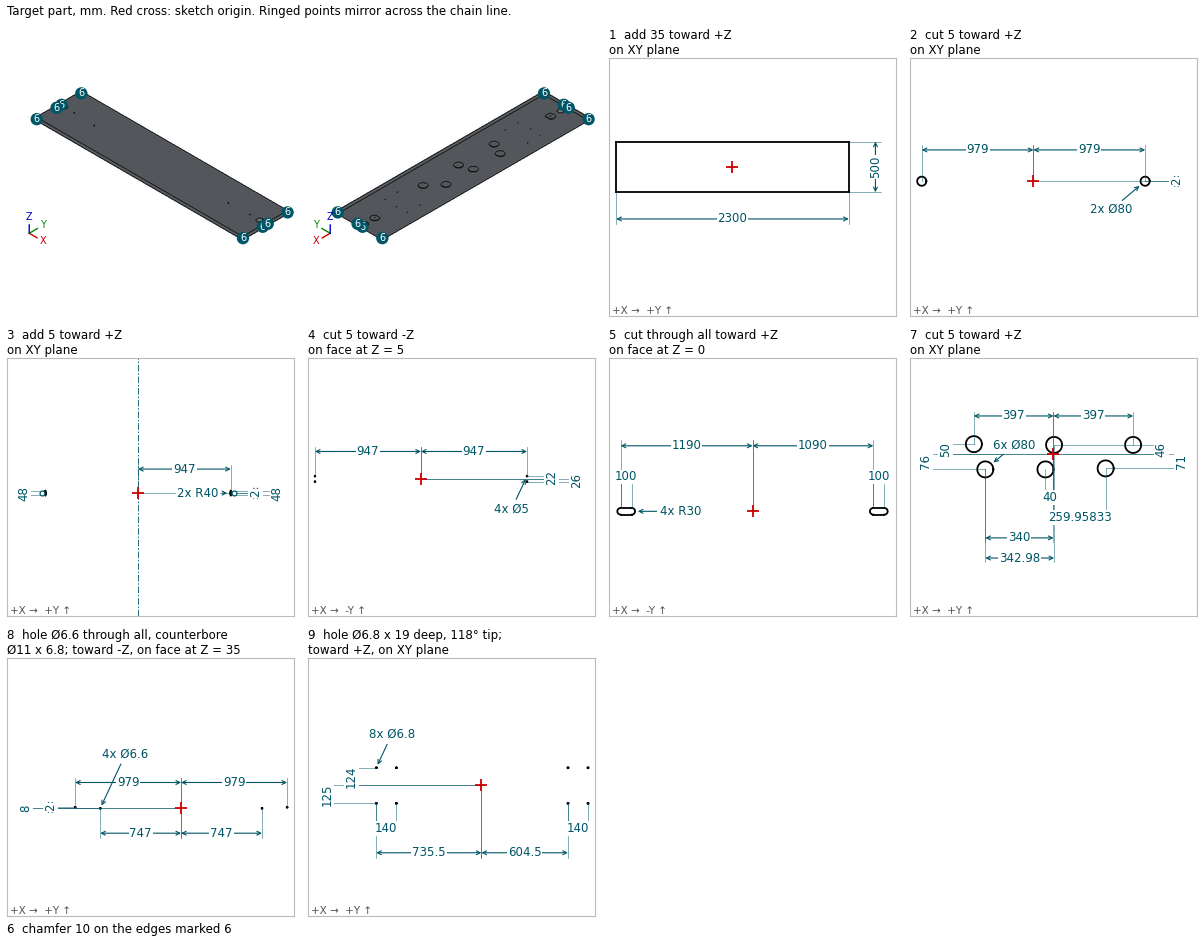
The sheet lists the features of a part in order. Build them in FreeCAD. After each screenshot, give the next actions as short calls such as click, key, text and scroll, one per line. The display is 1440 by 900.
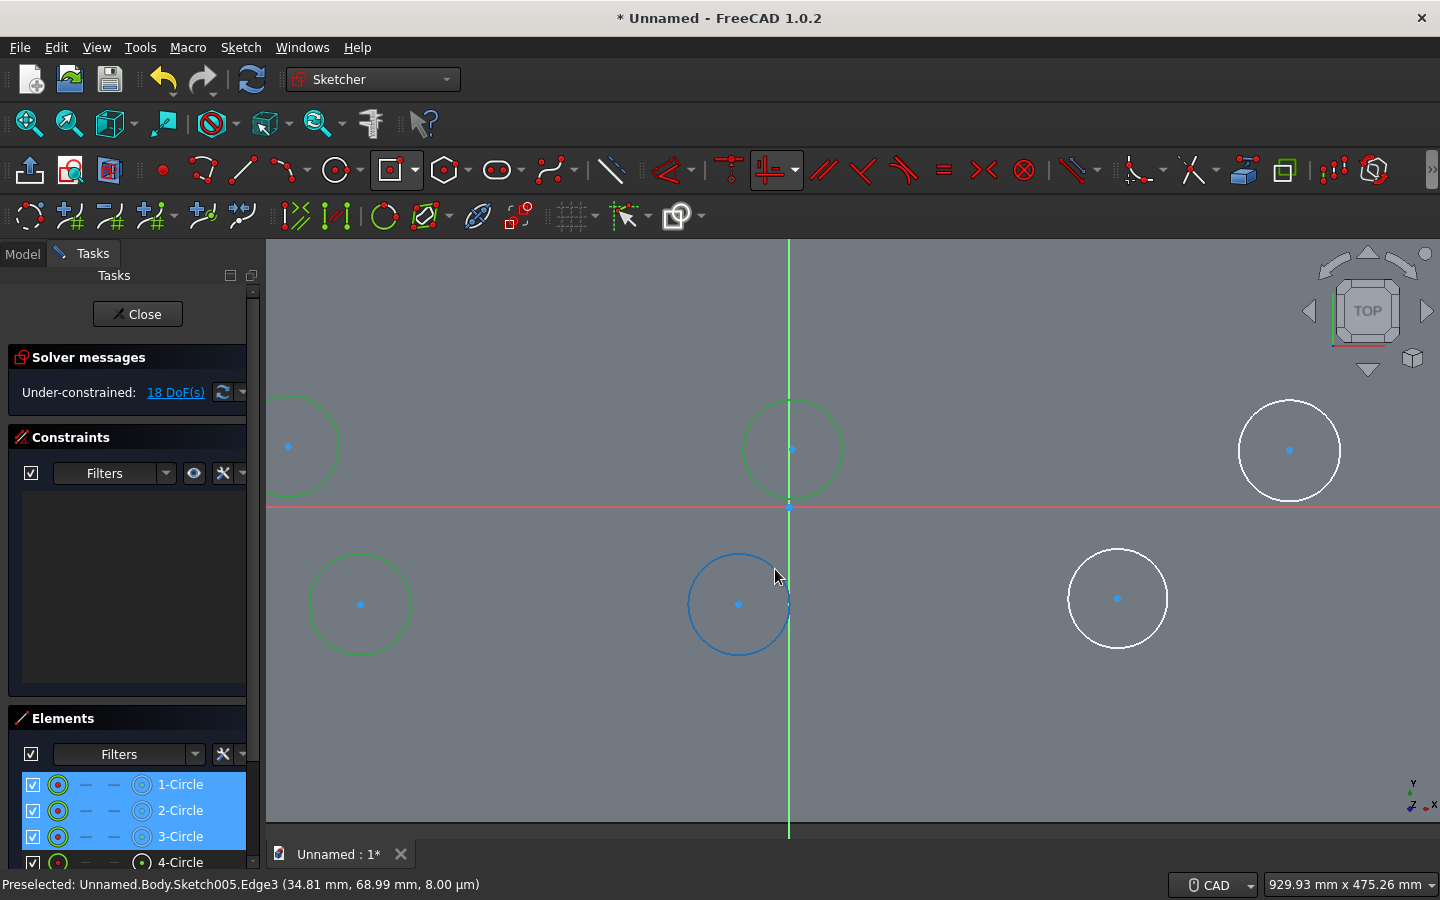
click(775, 569)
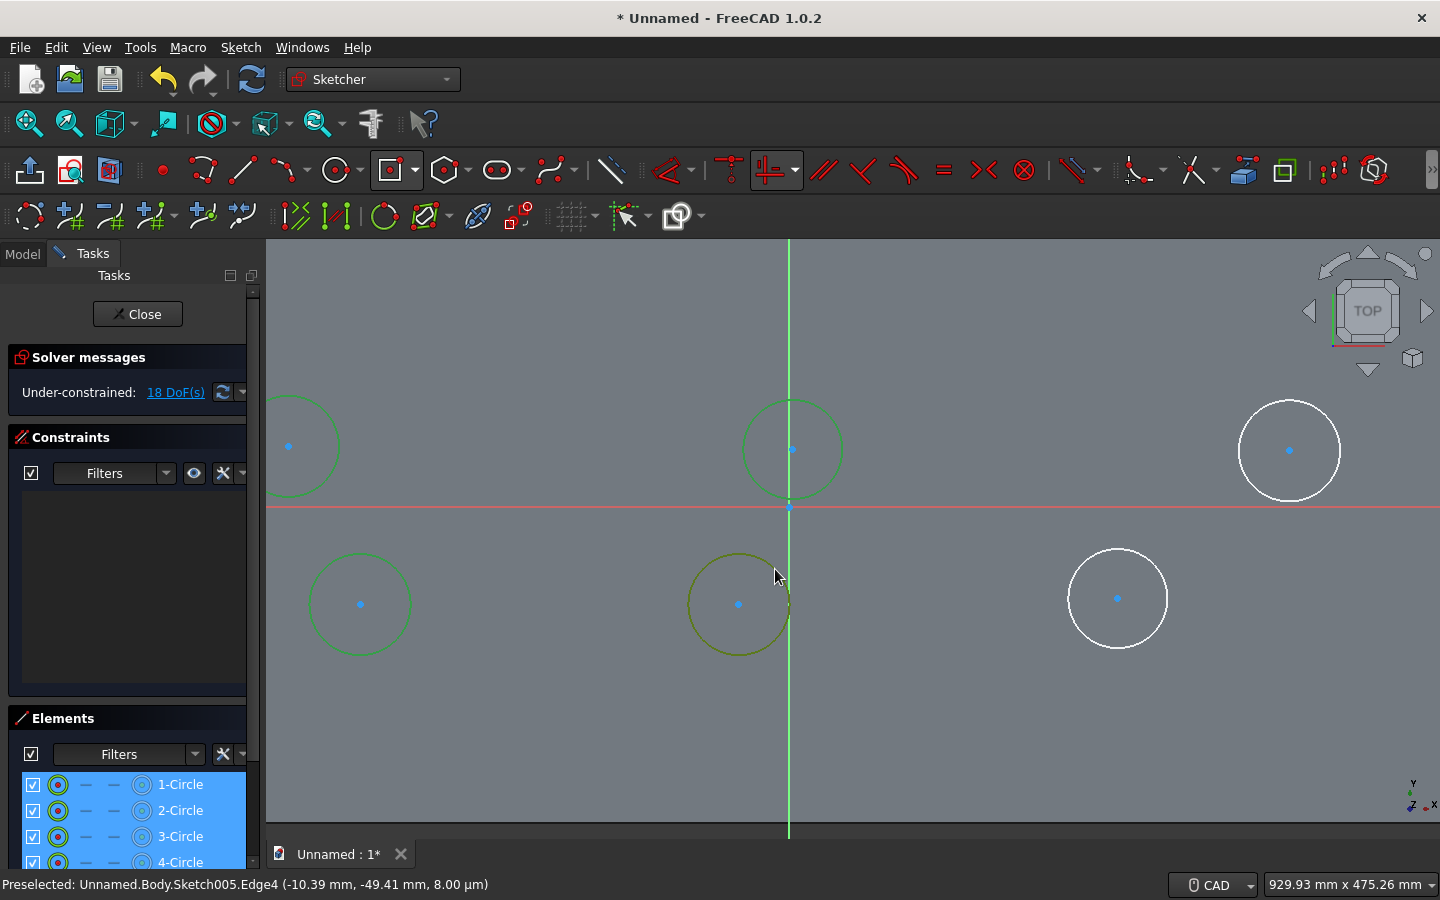
click(1153, 563)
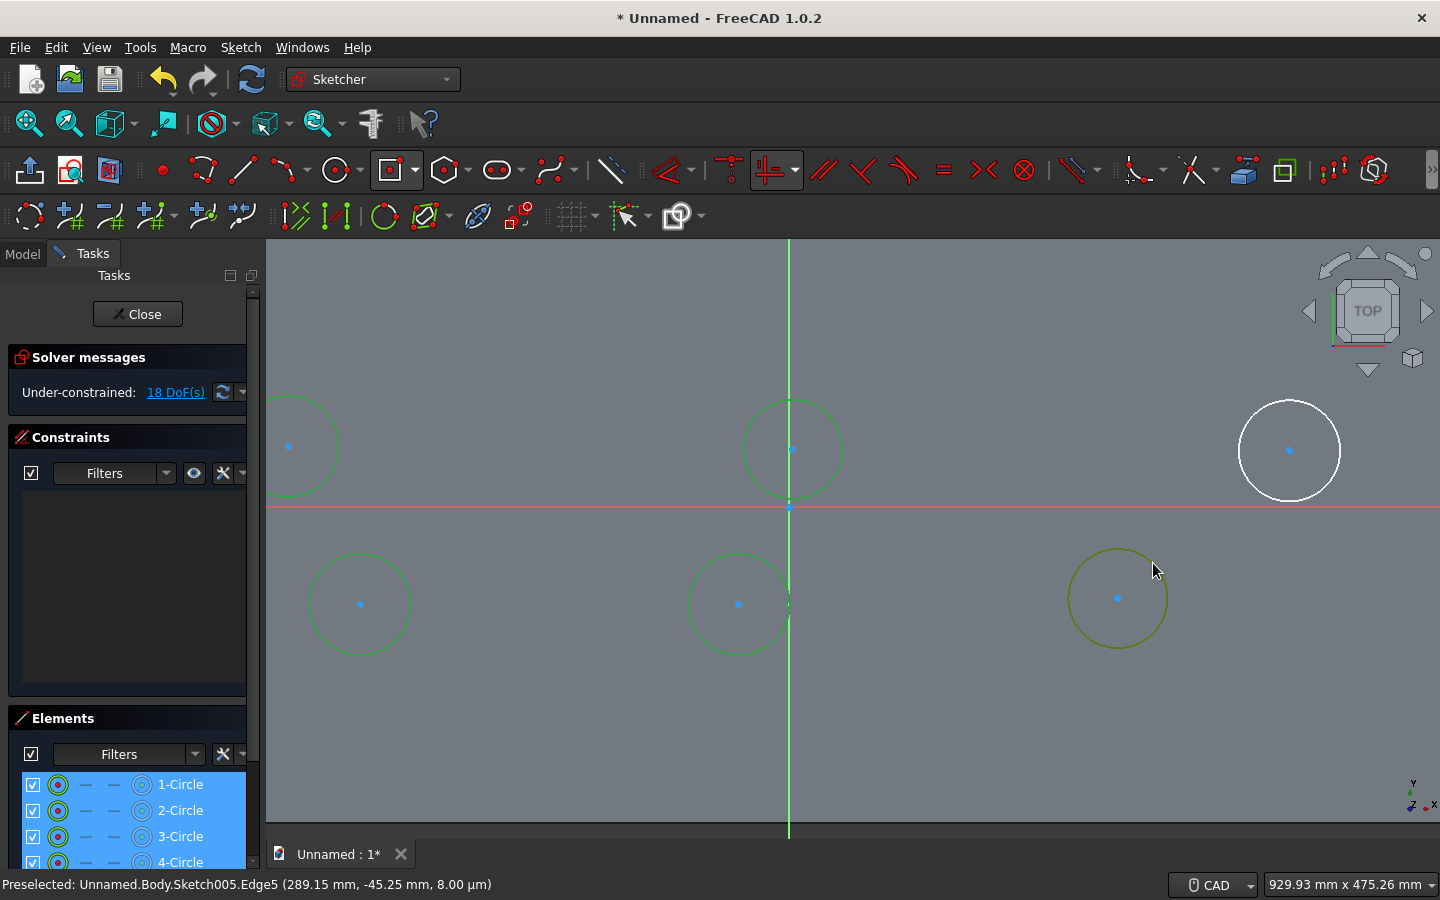
click(1254, 415)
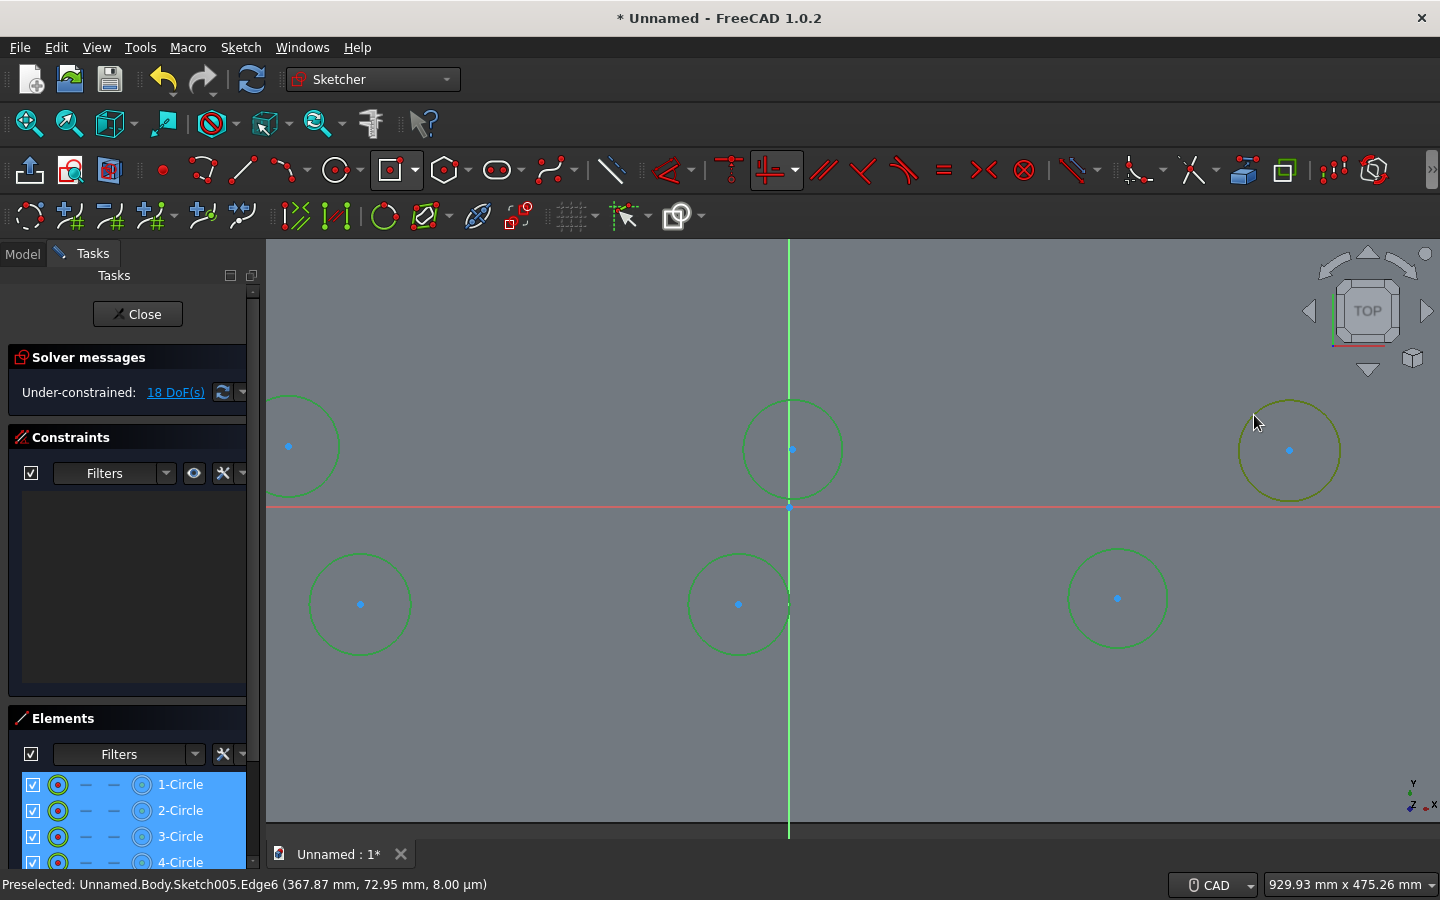
key(e)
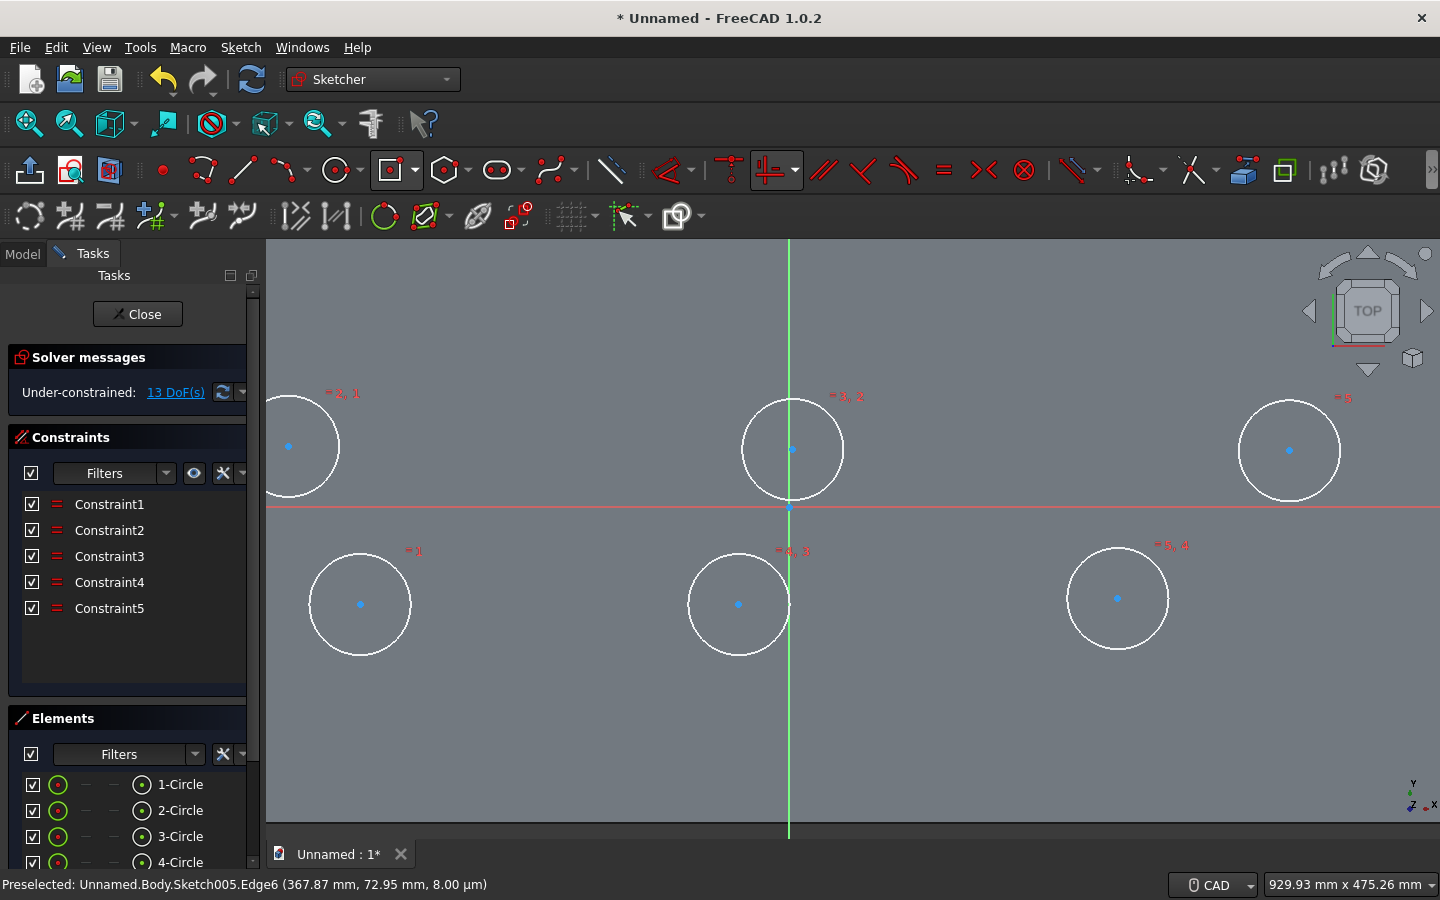
click(360, 605)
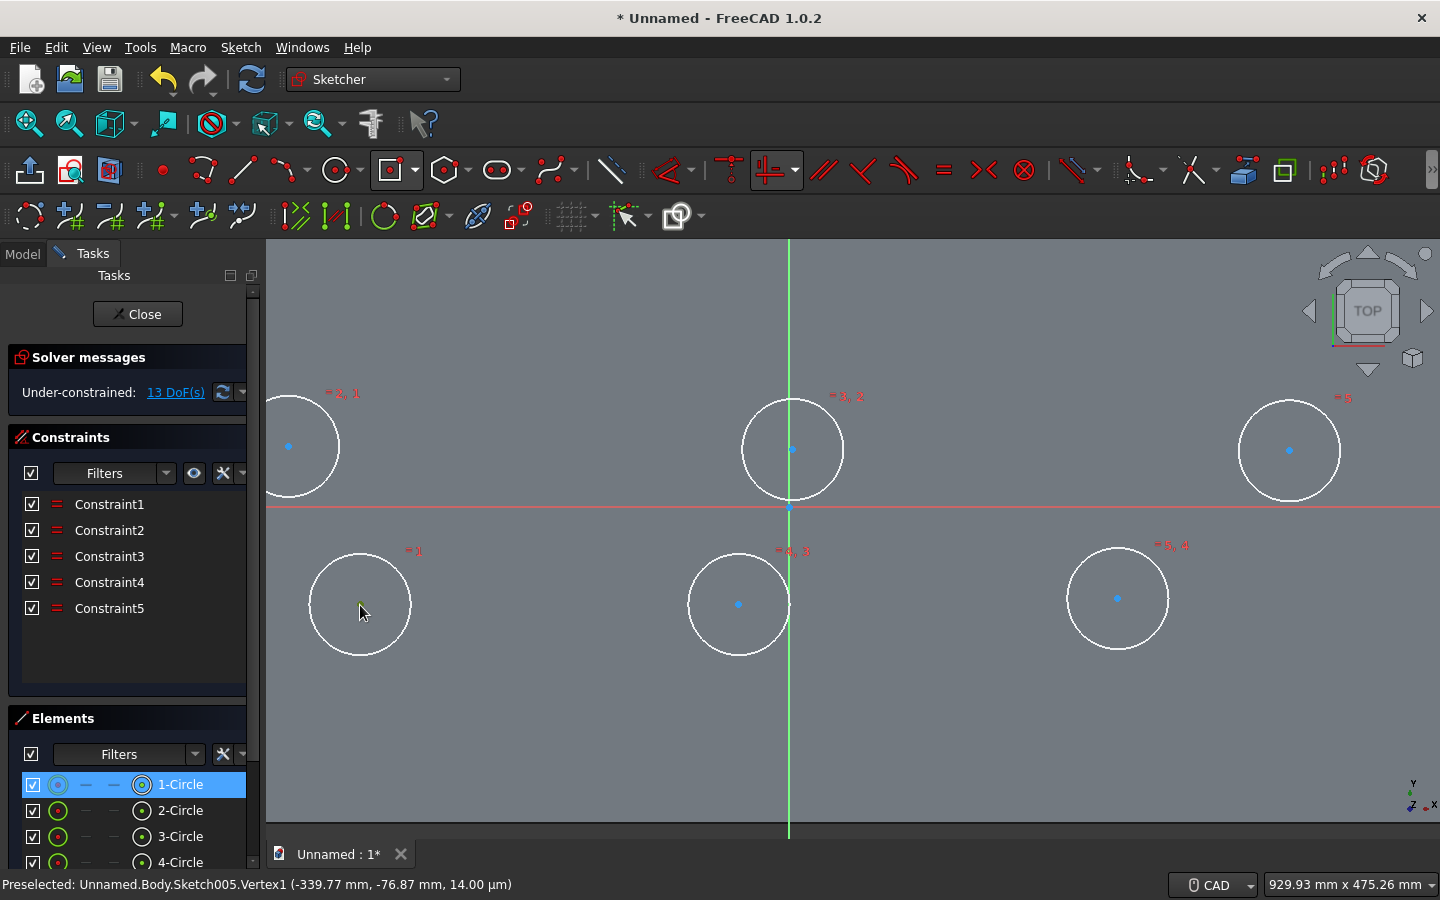
click(739, 605)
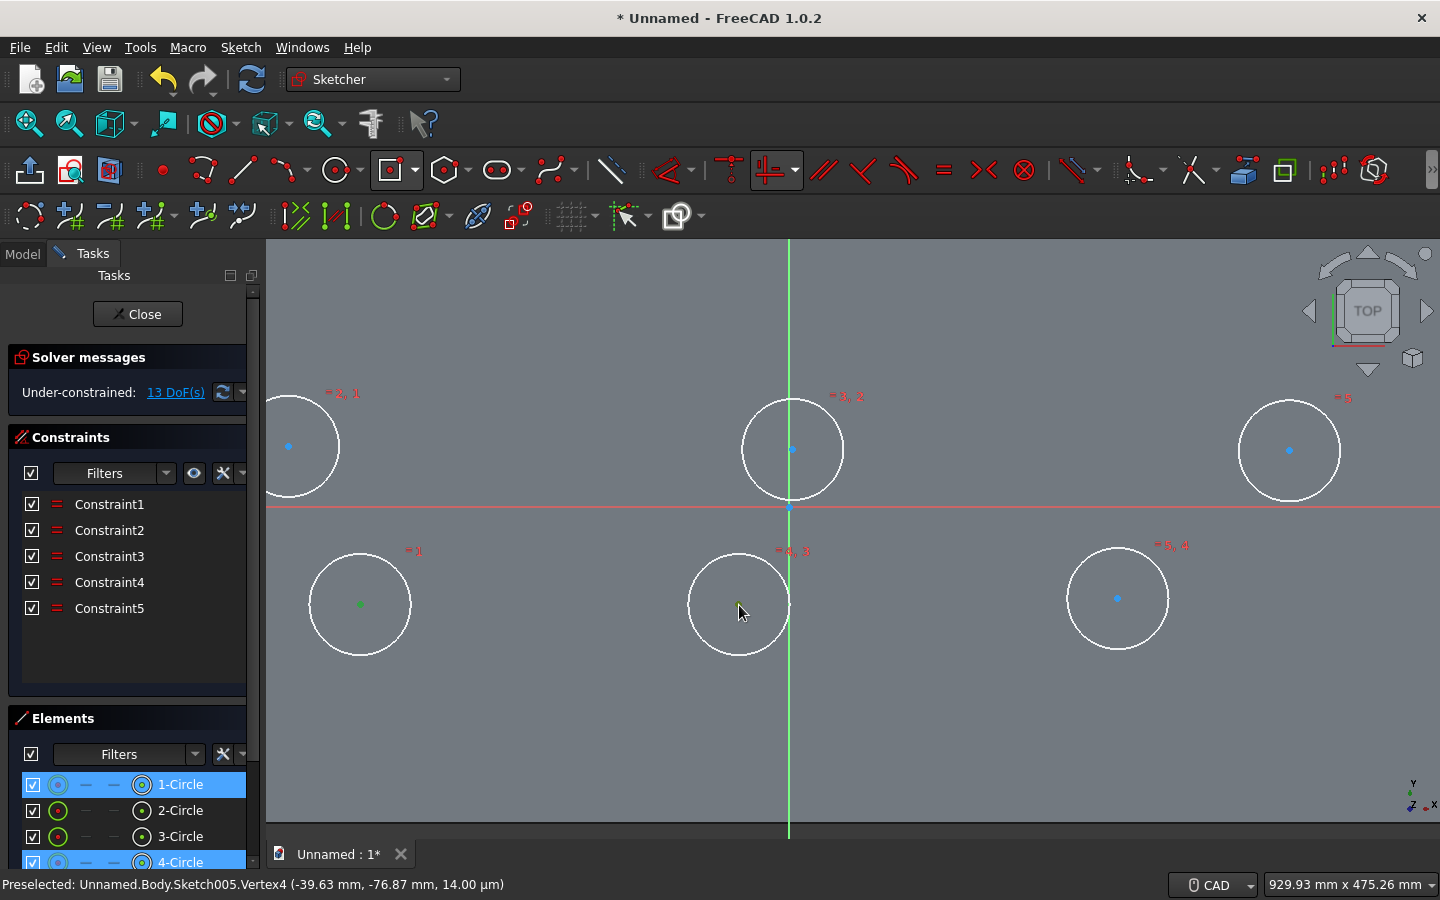
key(h)